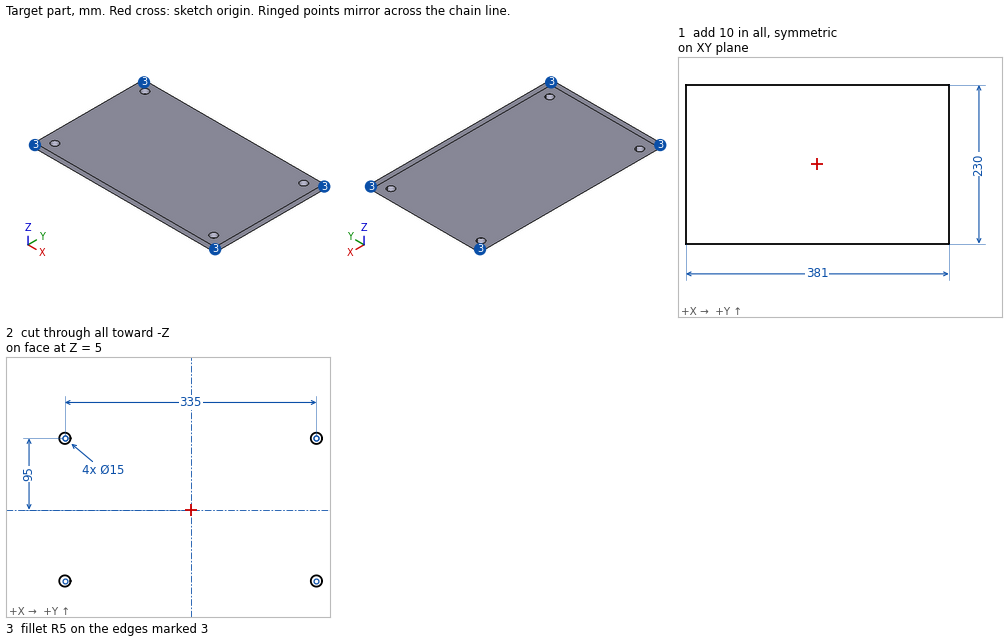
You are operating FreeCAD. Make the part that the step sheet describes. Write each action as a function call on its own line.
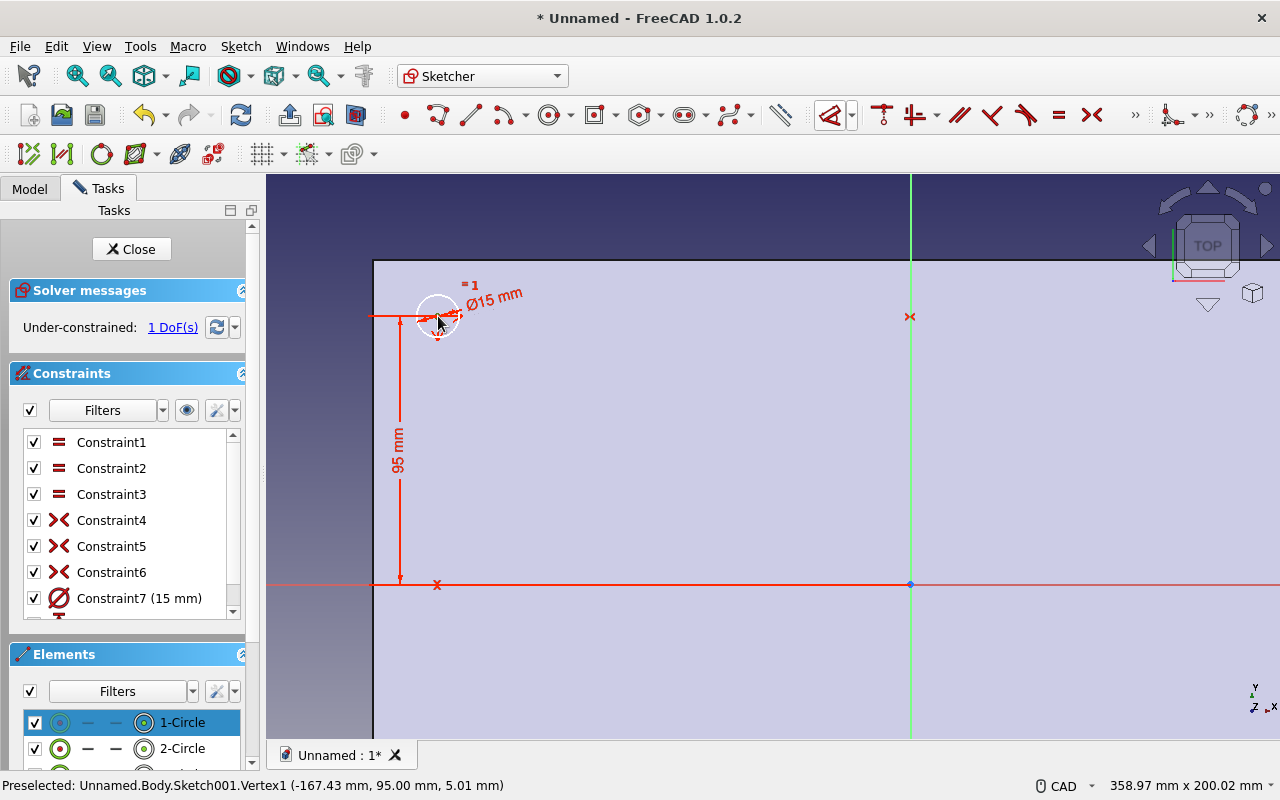
scroll(454, 301, down, 3)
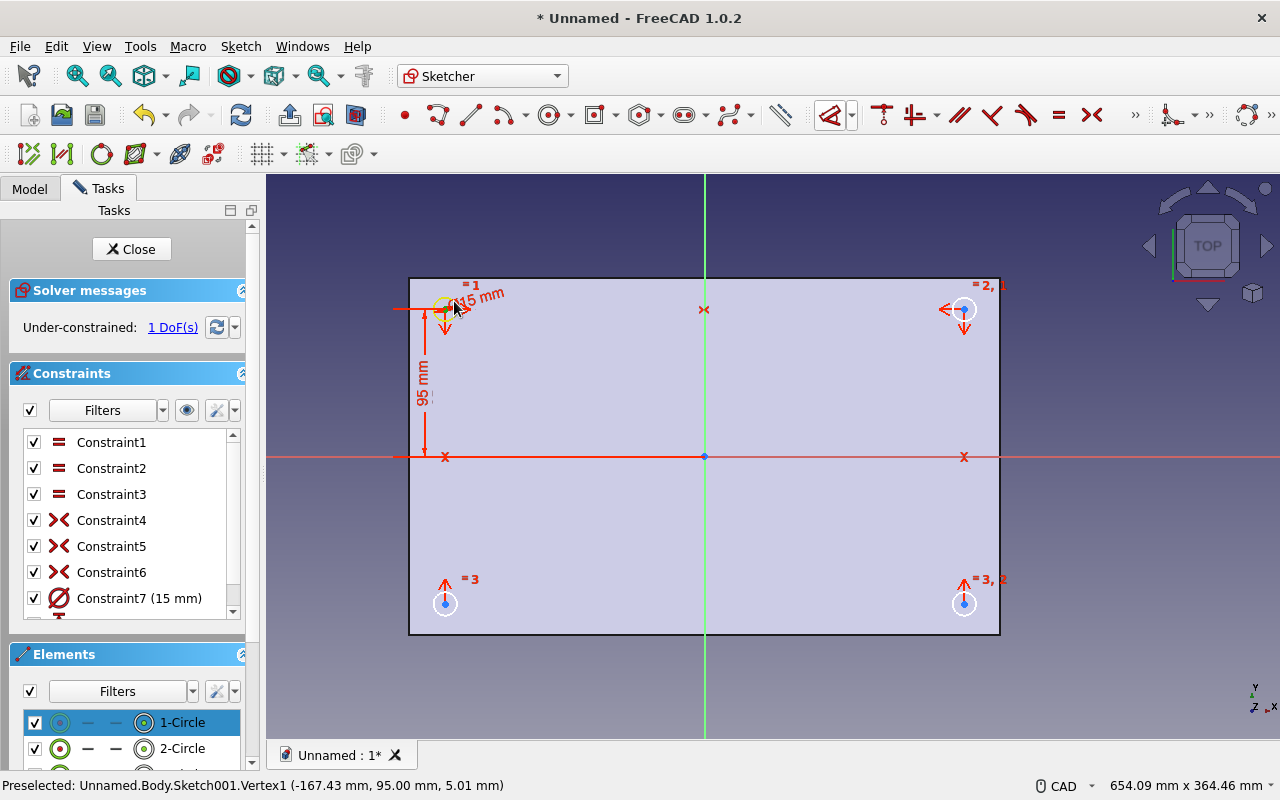
click(964, 309)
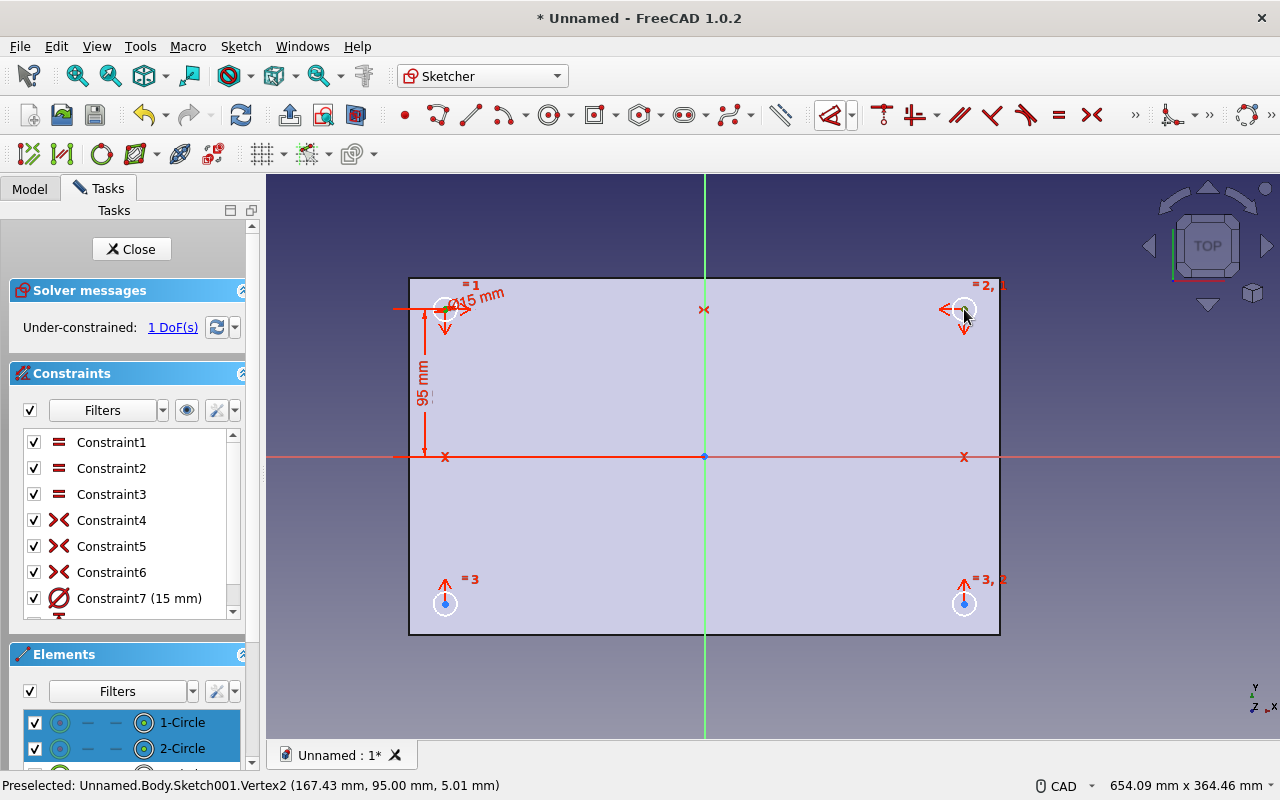
click(852, 116)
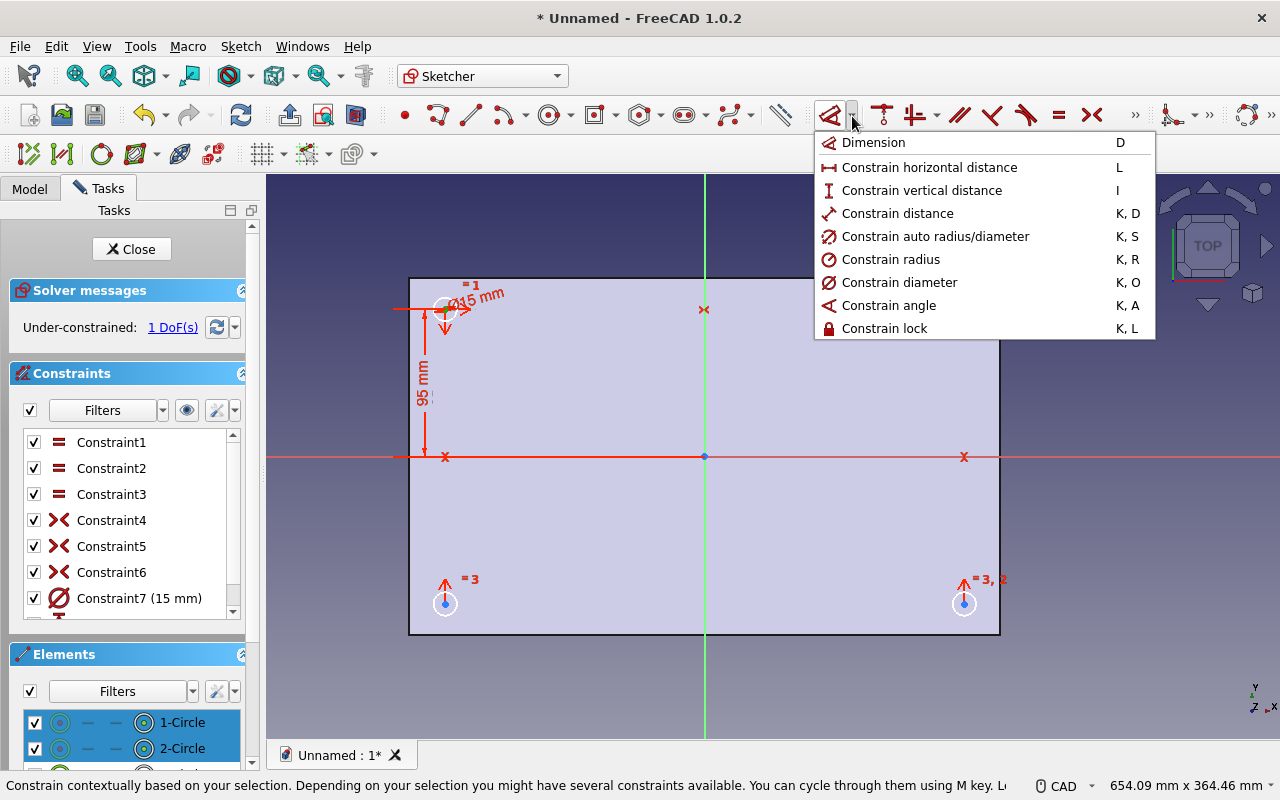
click(985, 168)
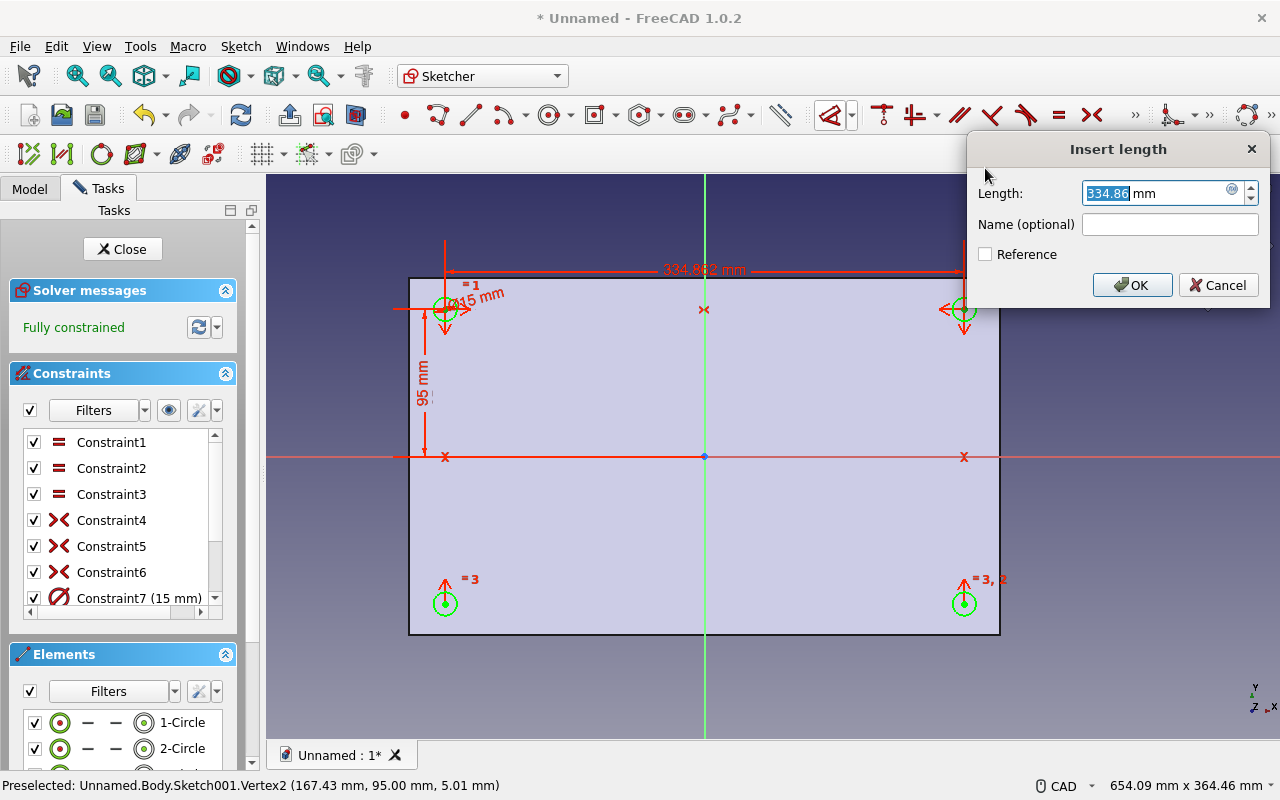
text(335)
key(Return)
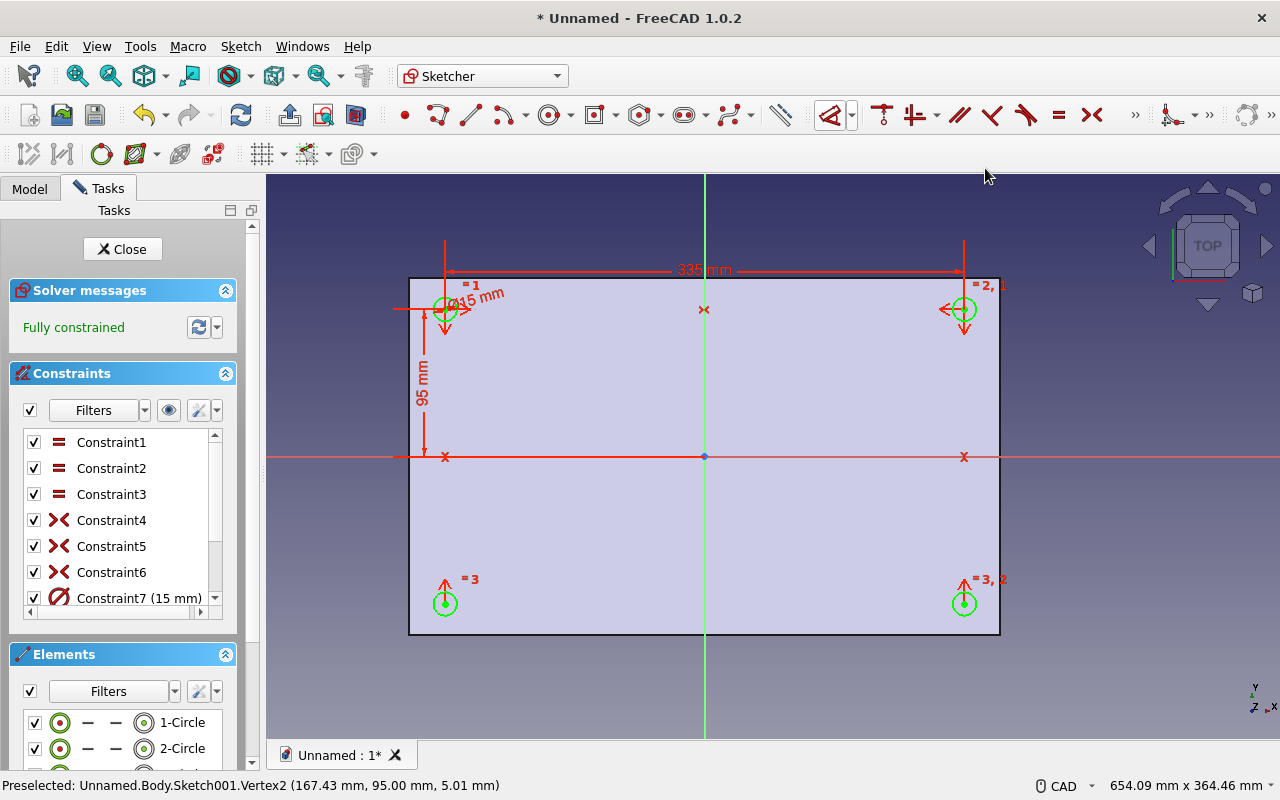
click(123, 249)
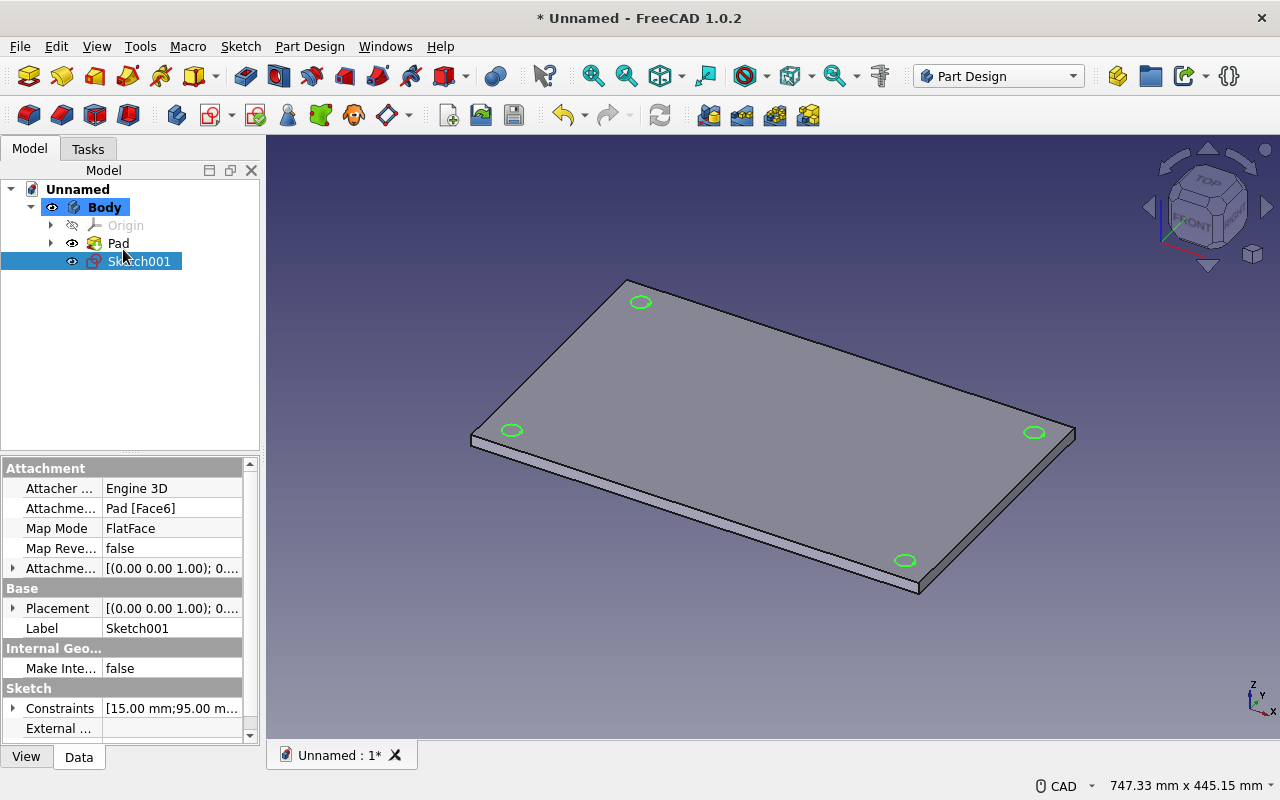
click(246, 76)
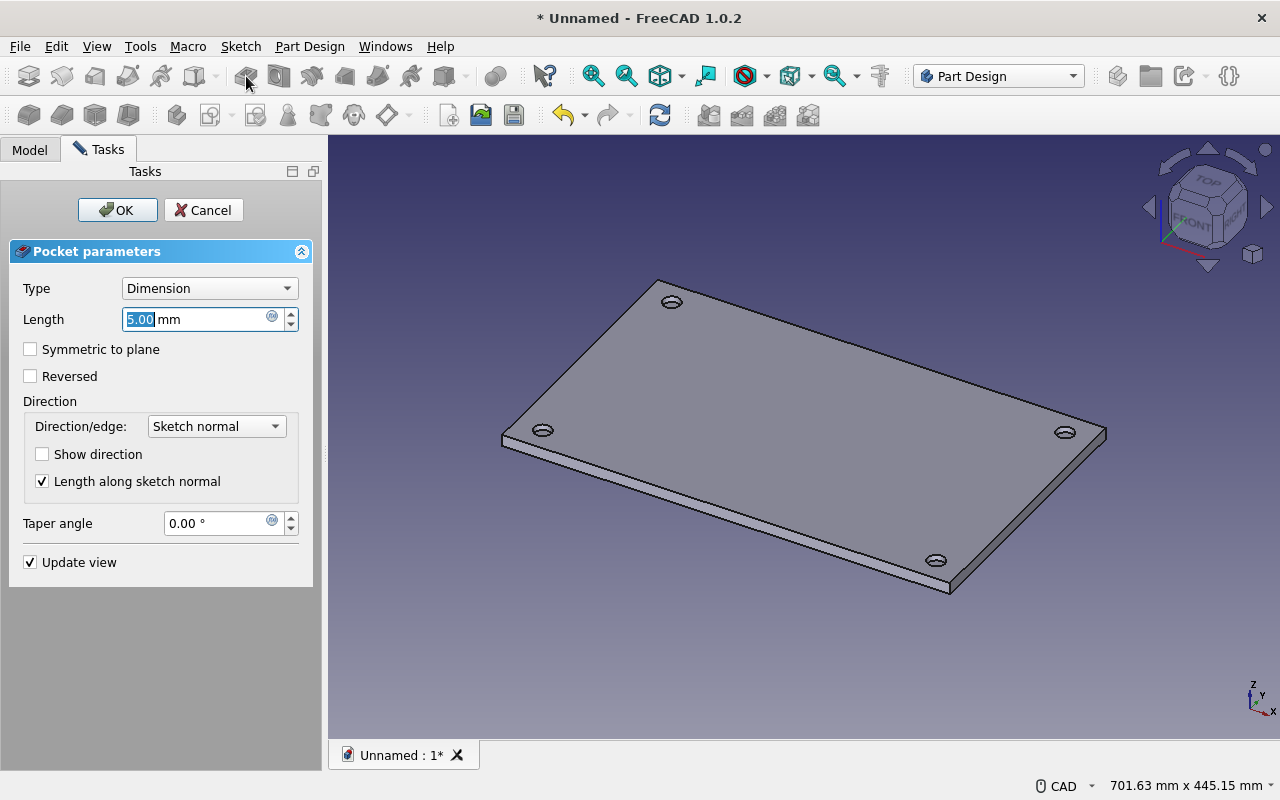
click(210, 288)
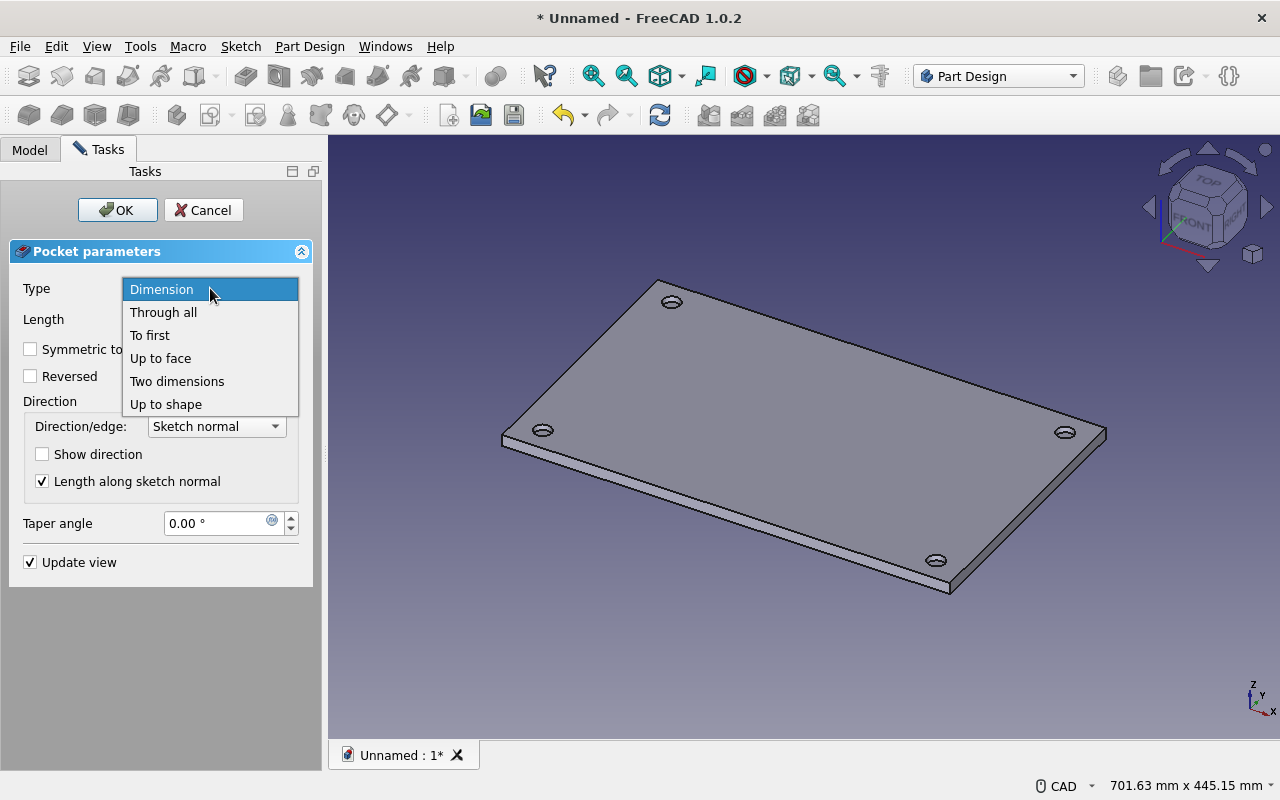
click(208, 312)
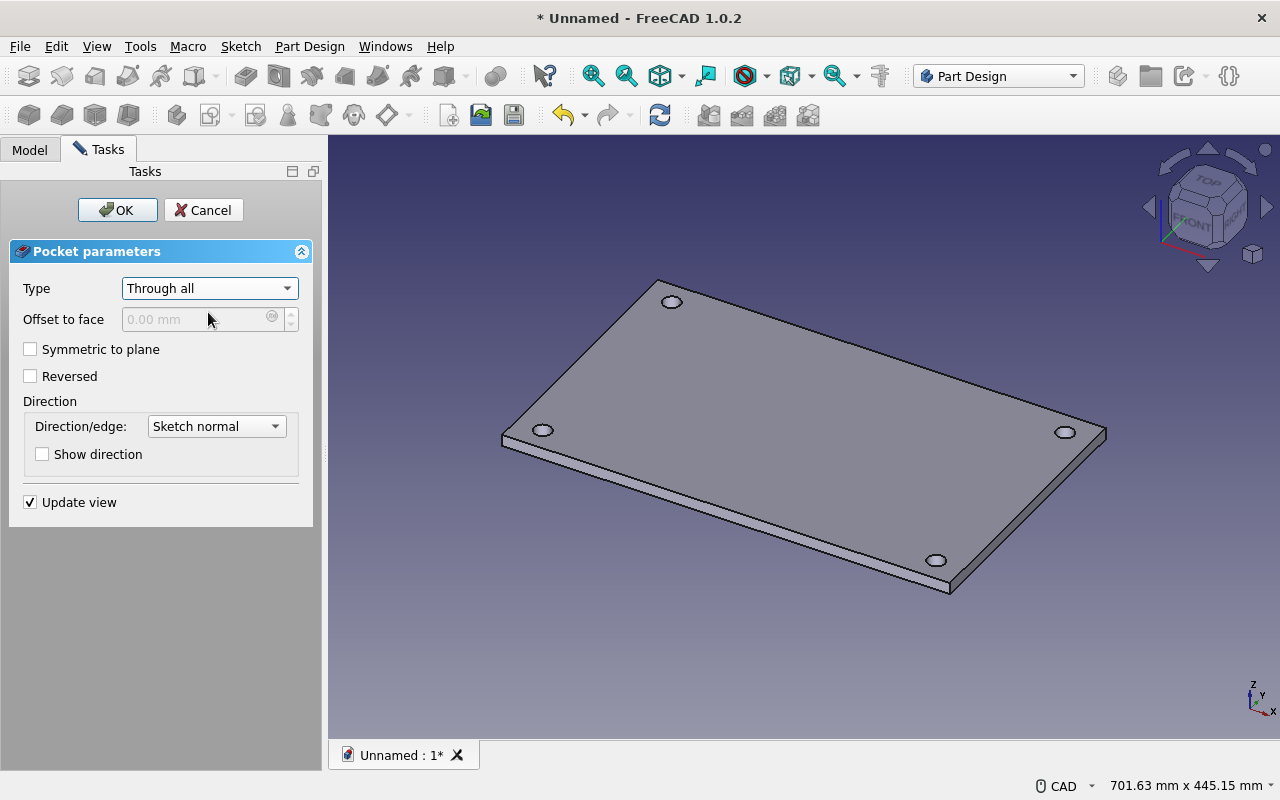
click(118, 210)